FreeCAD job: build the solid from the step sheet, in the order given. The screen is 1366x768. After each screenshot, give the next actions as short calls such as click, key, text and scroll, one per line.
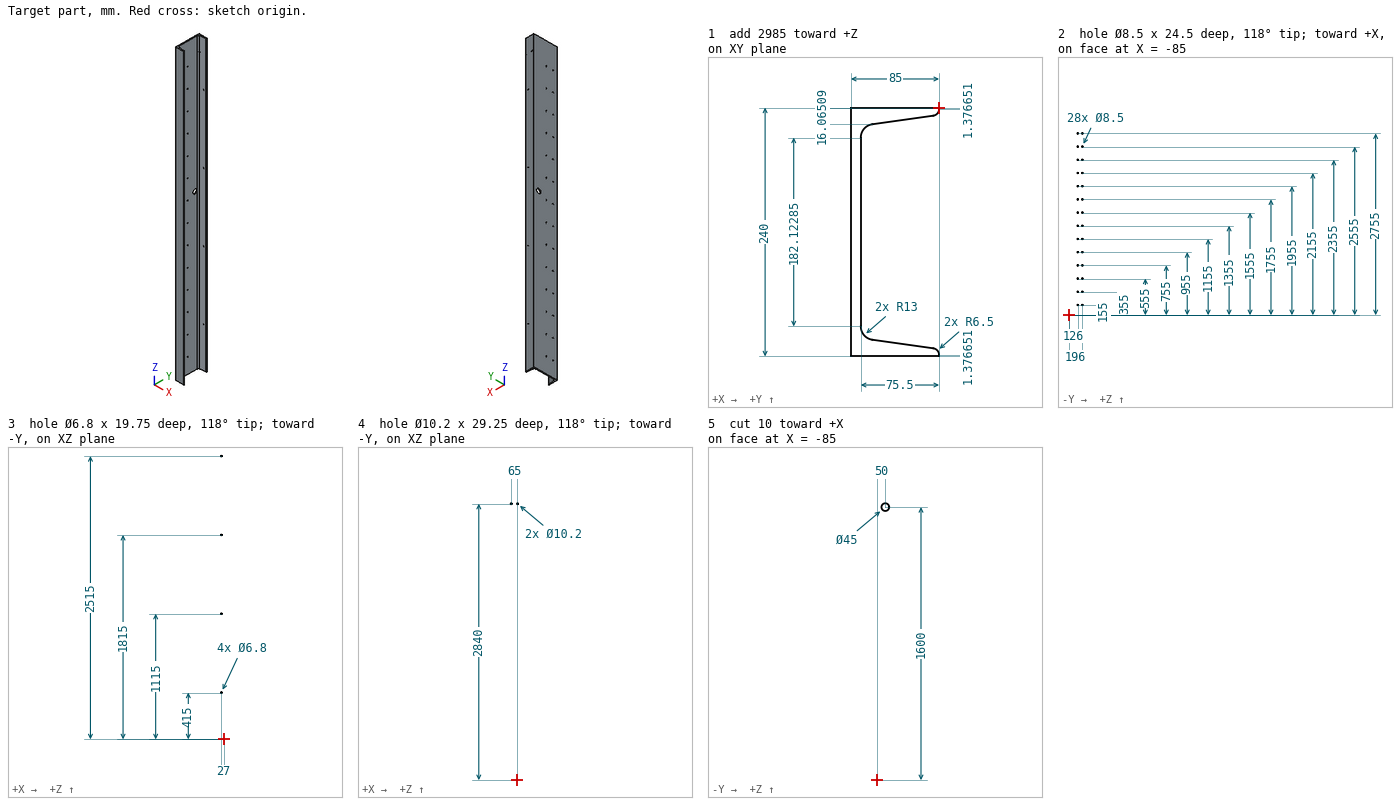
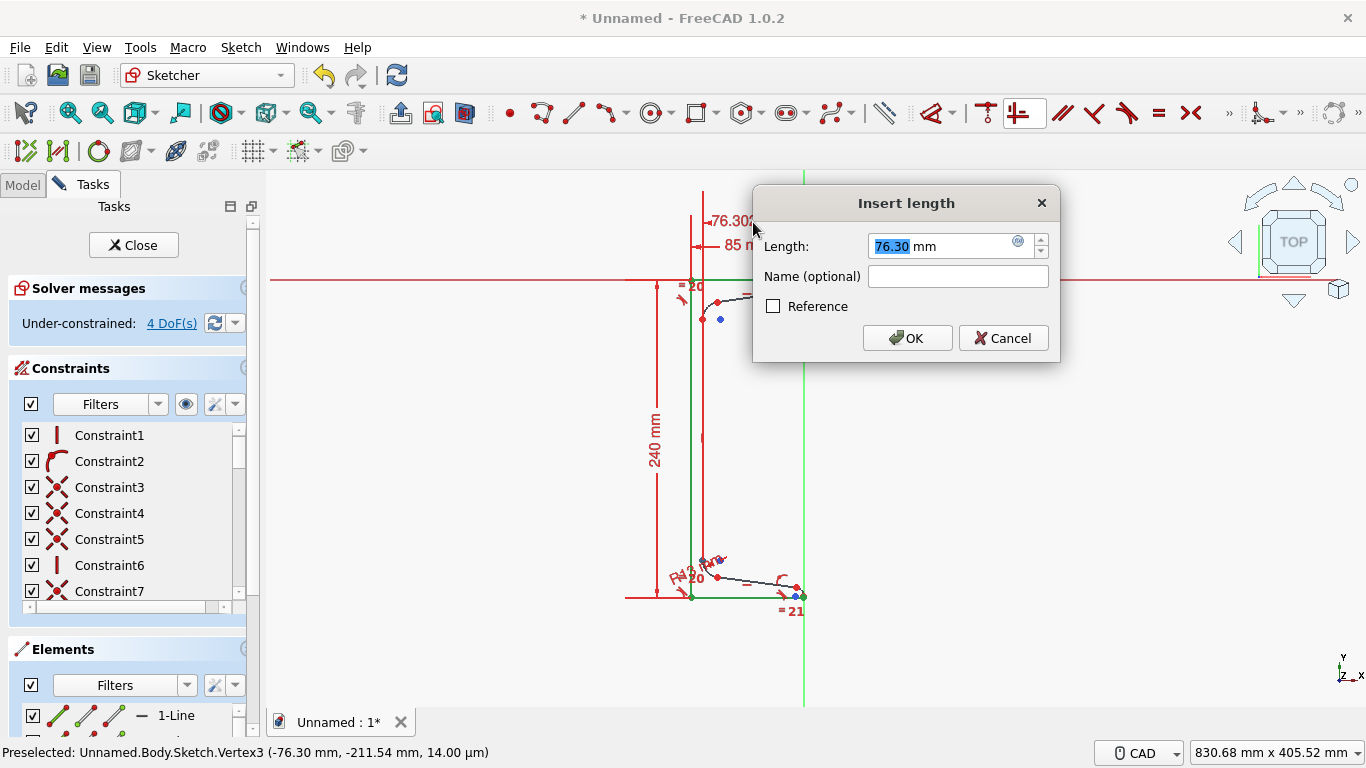
text(75.5)
key(Return)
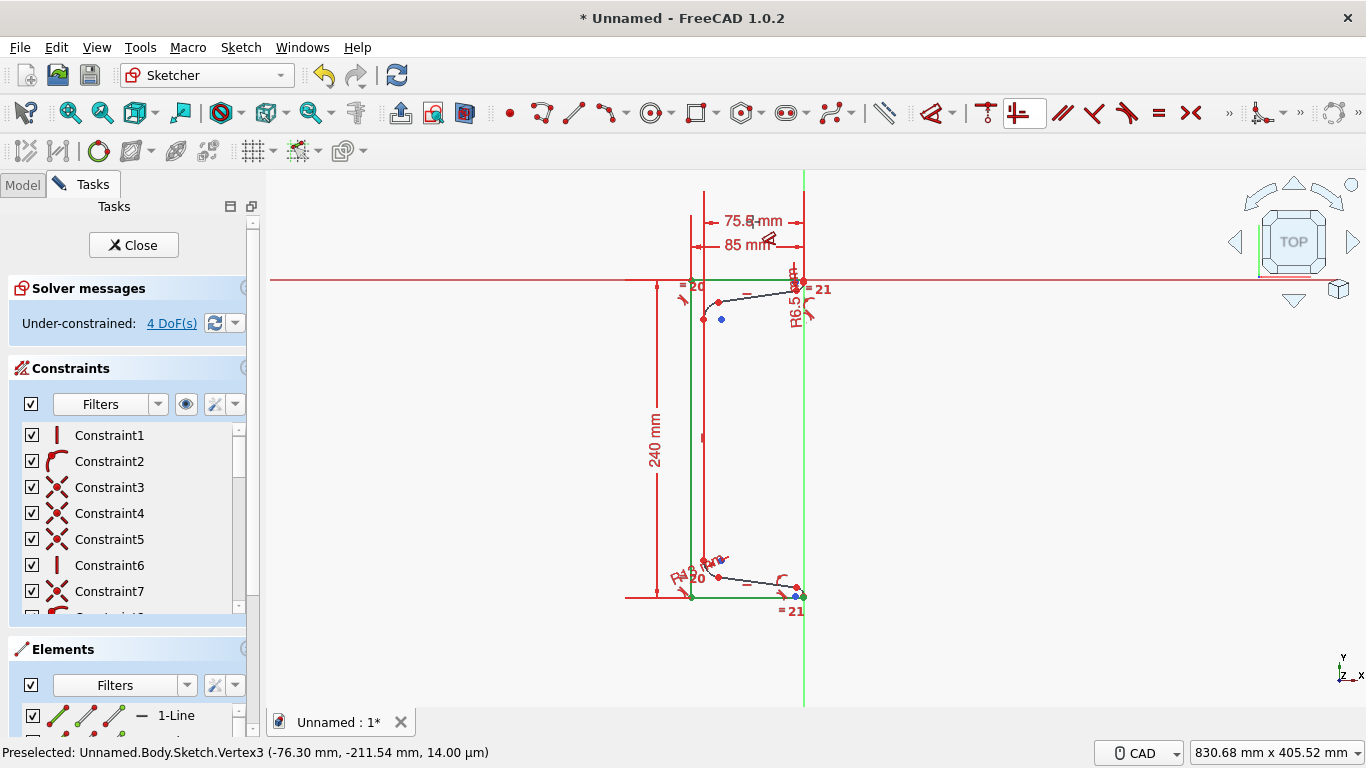
scroll(804, 281, up, 16)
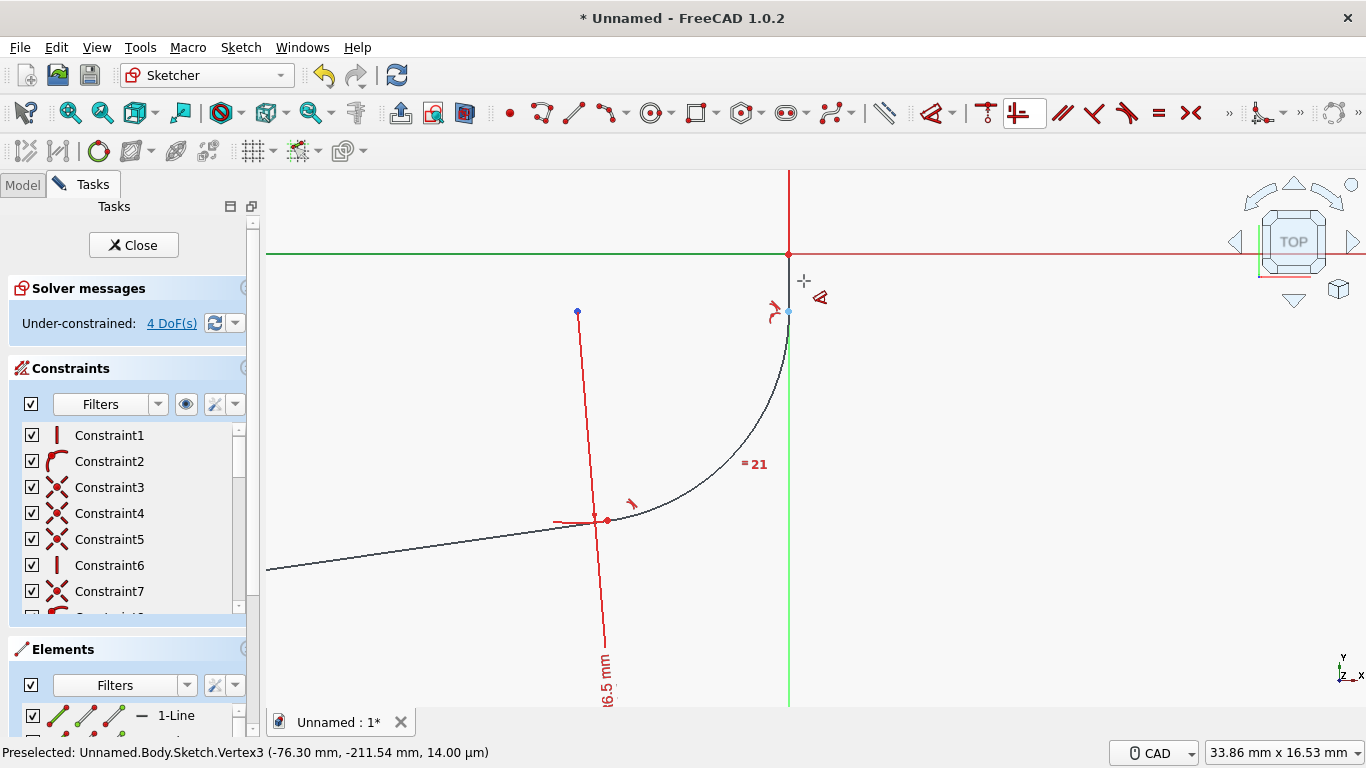
click(789, 283)
click(823, 283)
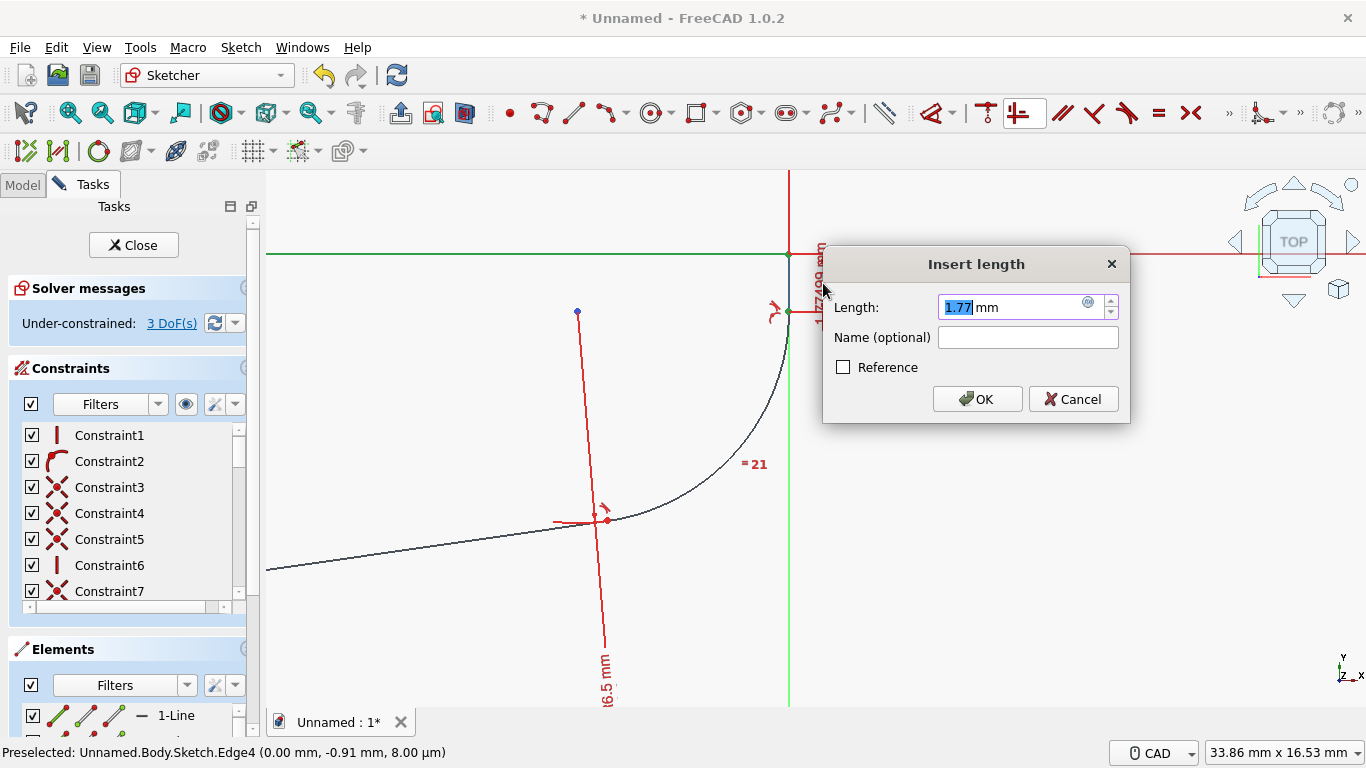
text(1.376651)
key(Return)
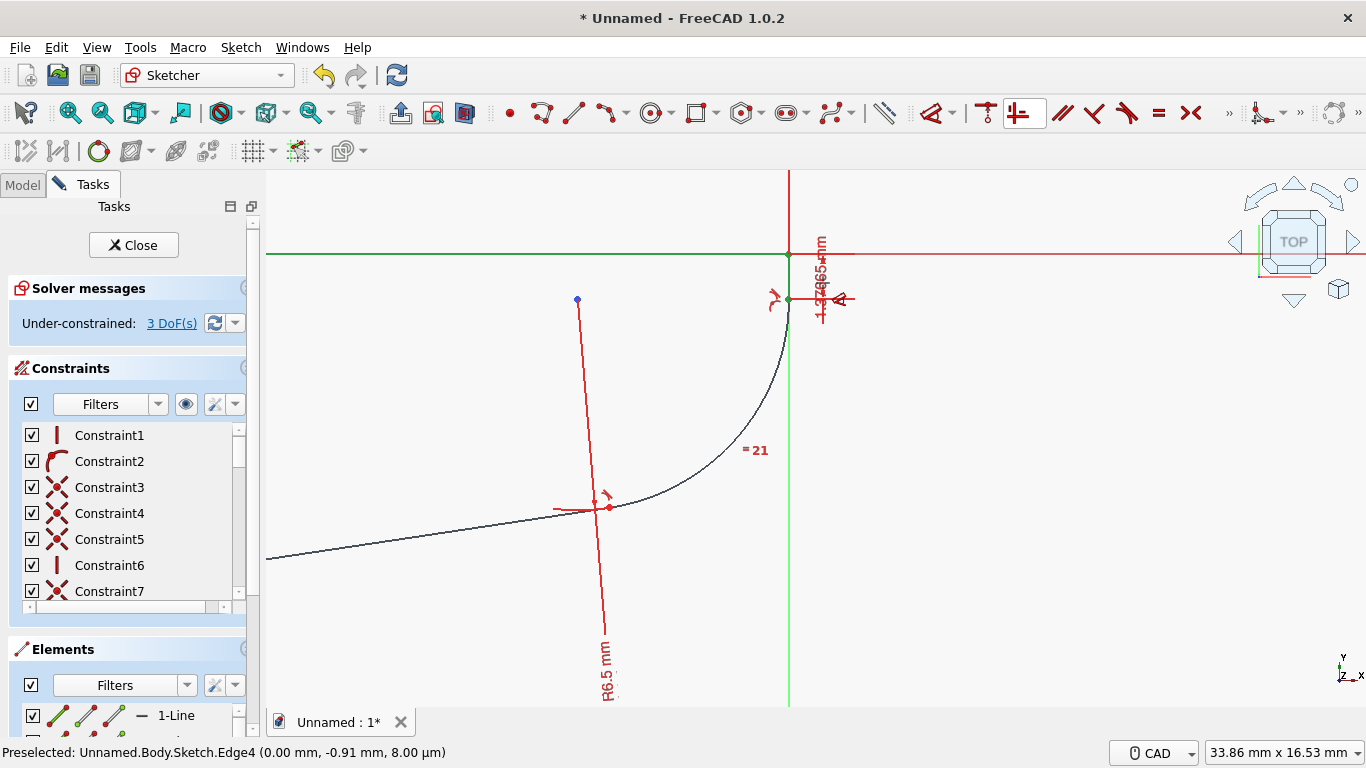
scroll(818, 244, down, 15)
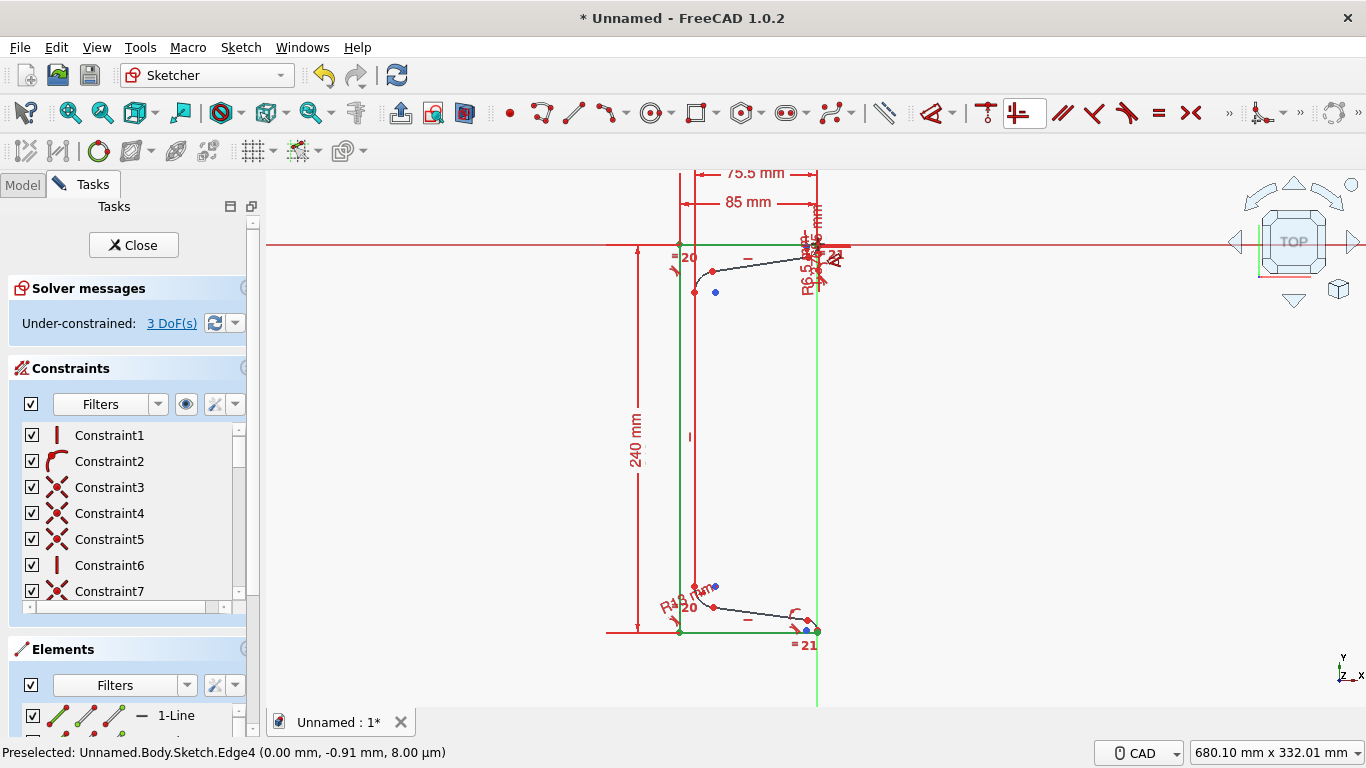
scroll(817, 632, up, 15)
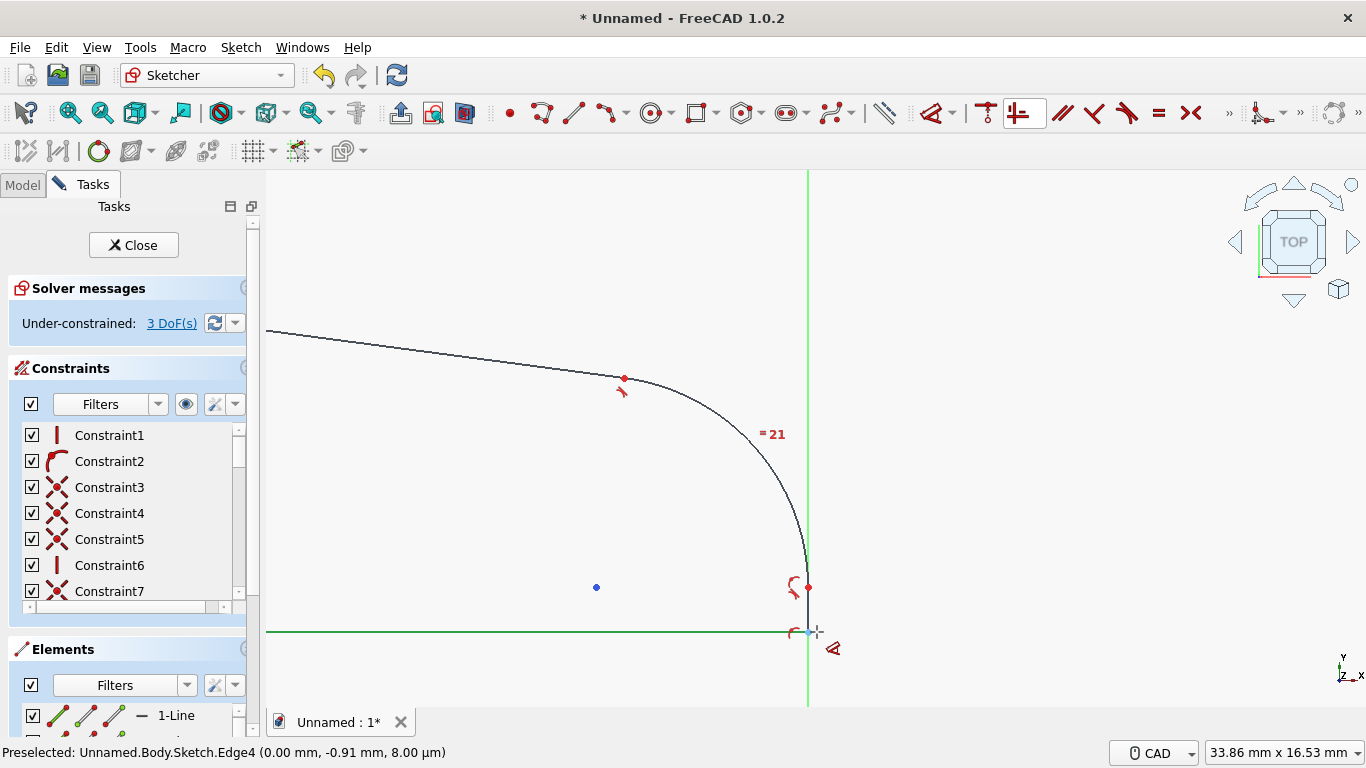
click(808, 619)
click(842, 610)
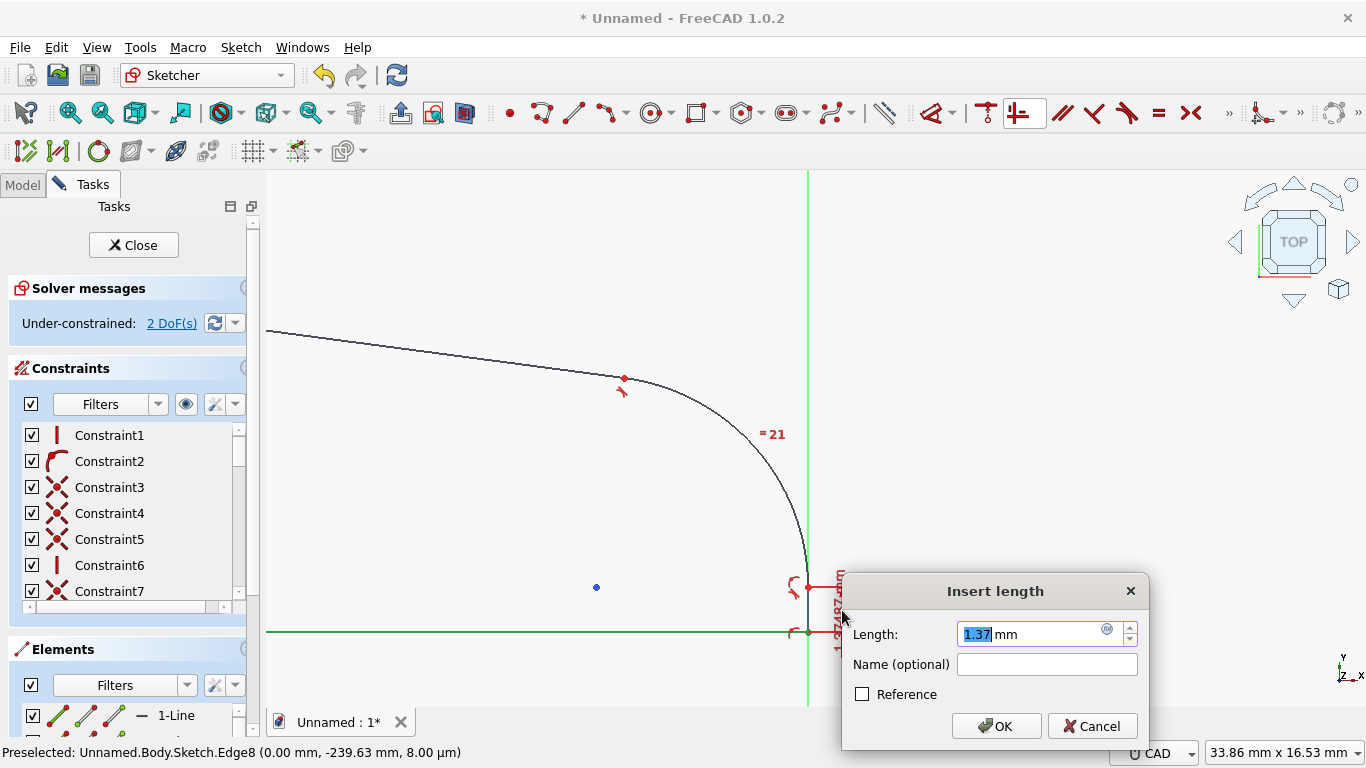
text(1.376651)
key(Return)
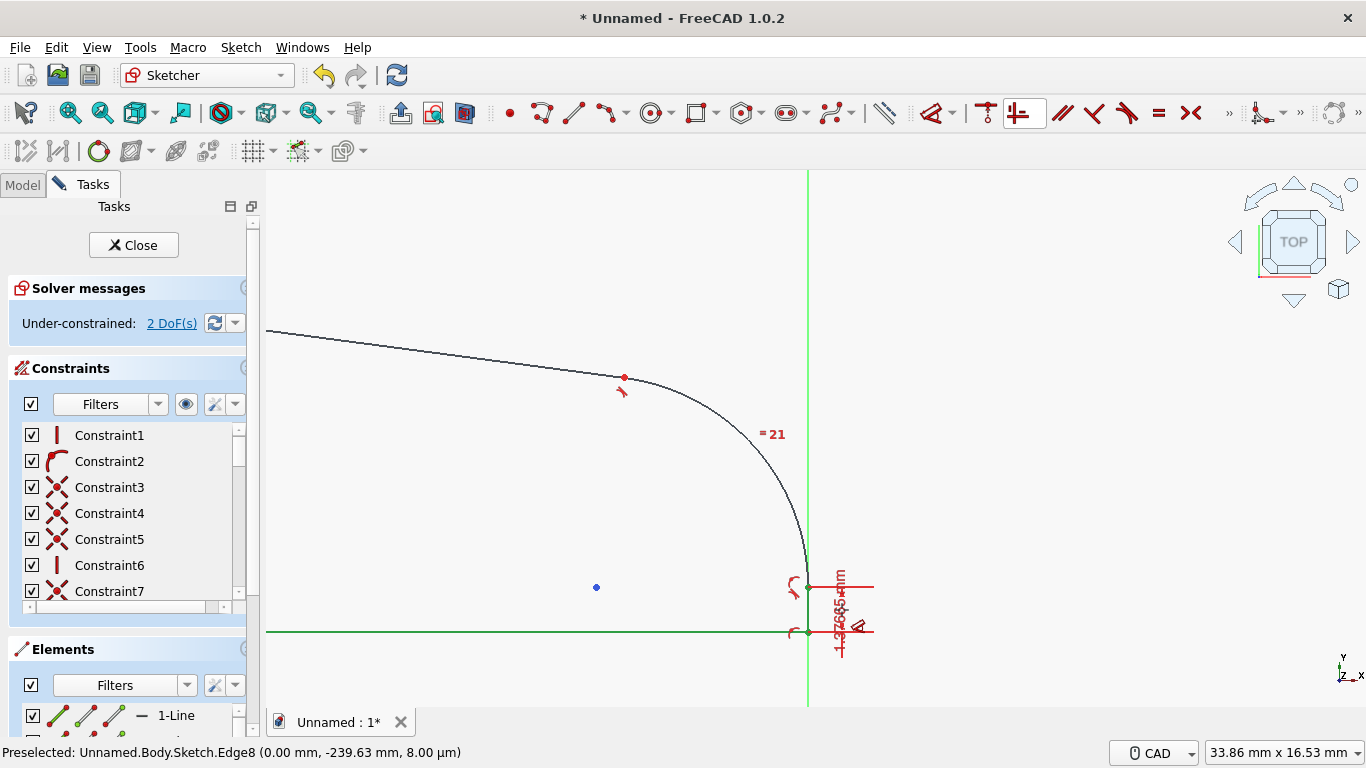
scroll(817, 633, down, 15)